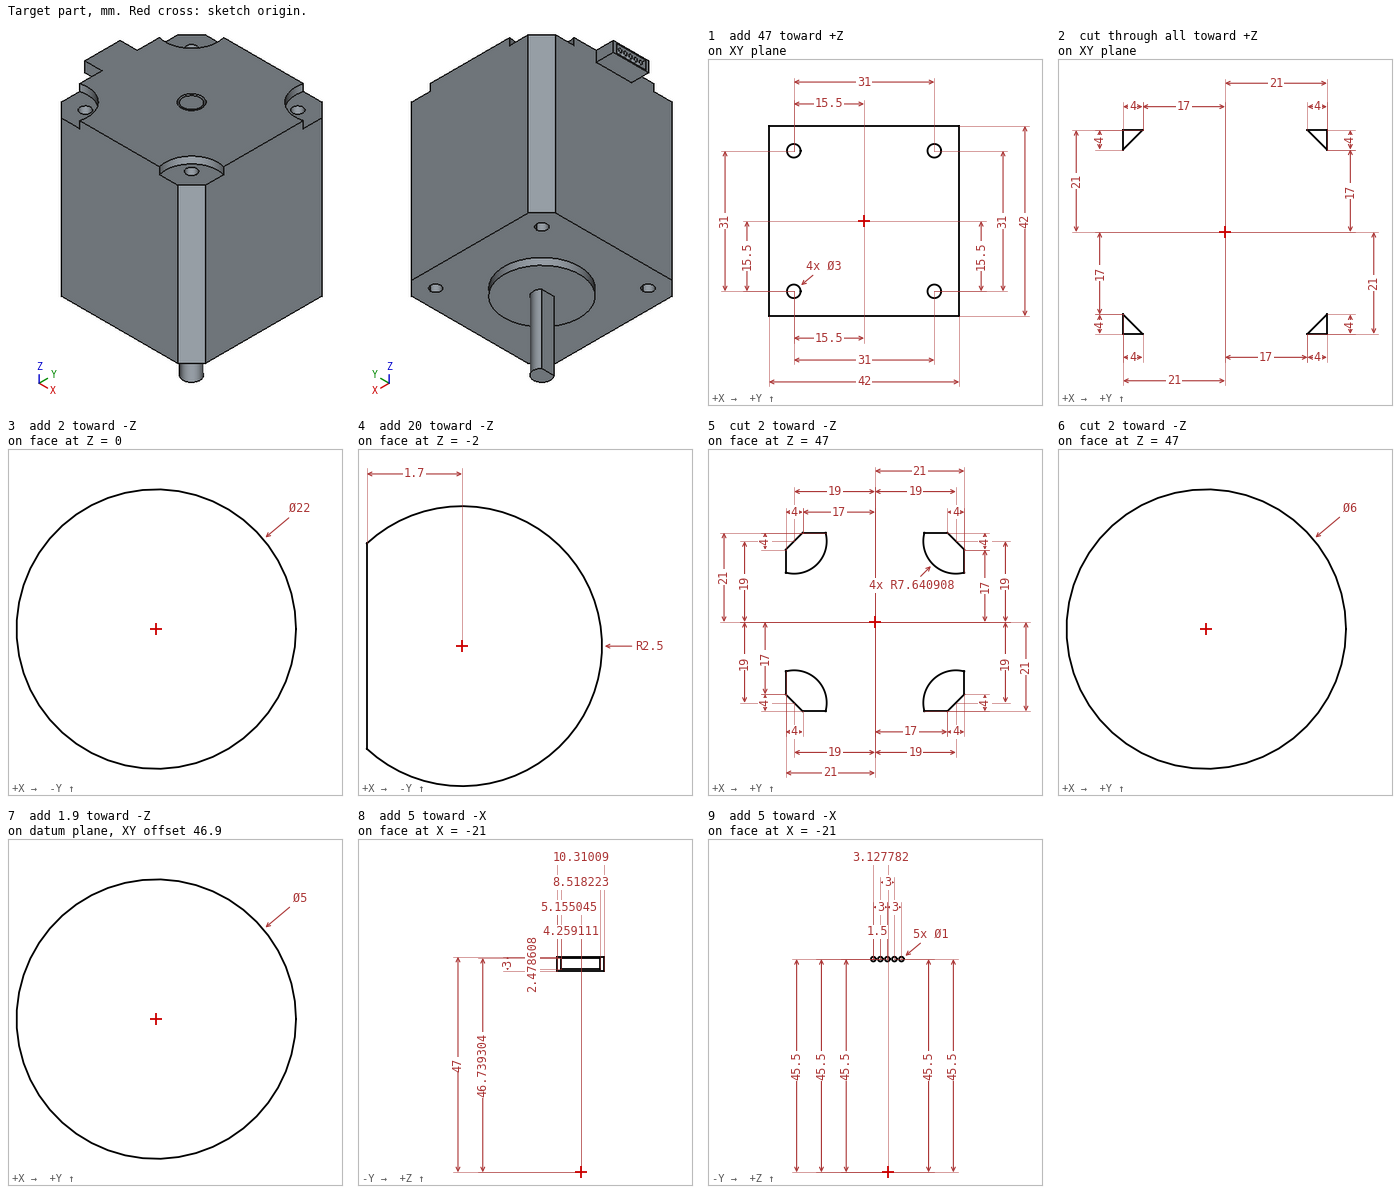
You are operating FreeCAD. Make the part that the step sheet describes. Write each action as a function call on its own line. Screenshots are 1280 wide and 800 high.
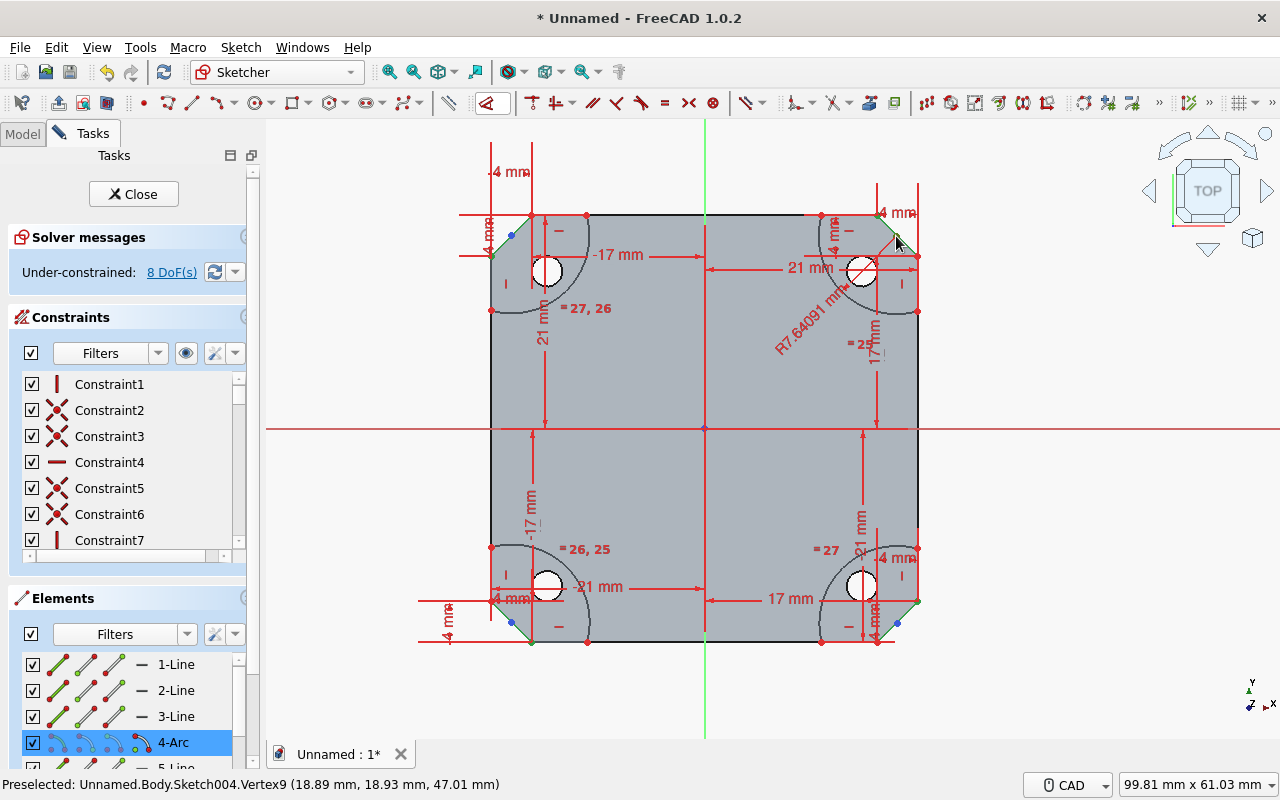
click(504, 104)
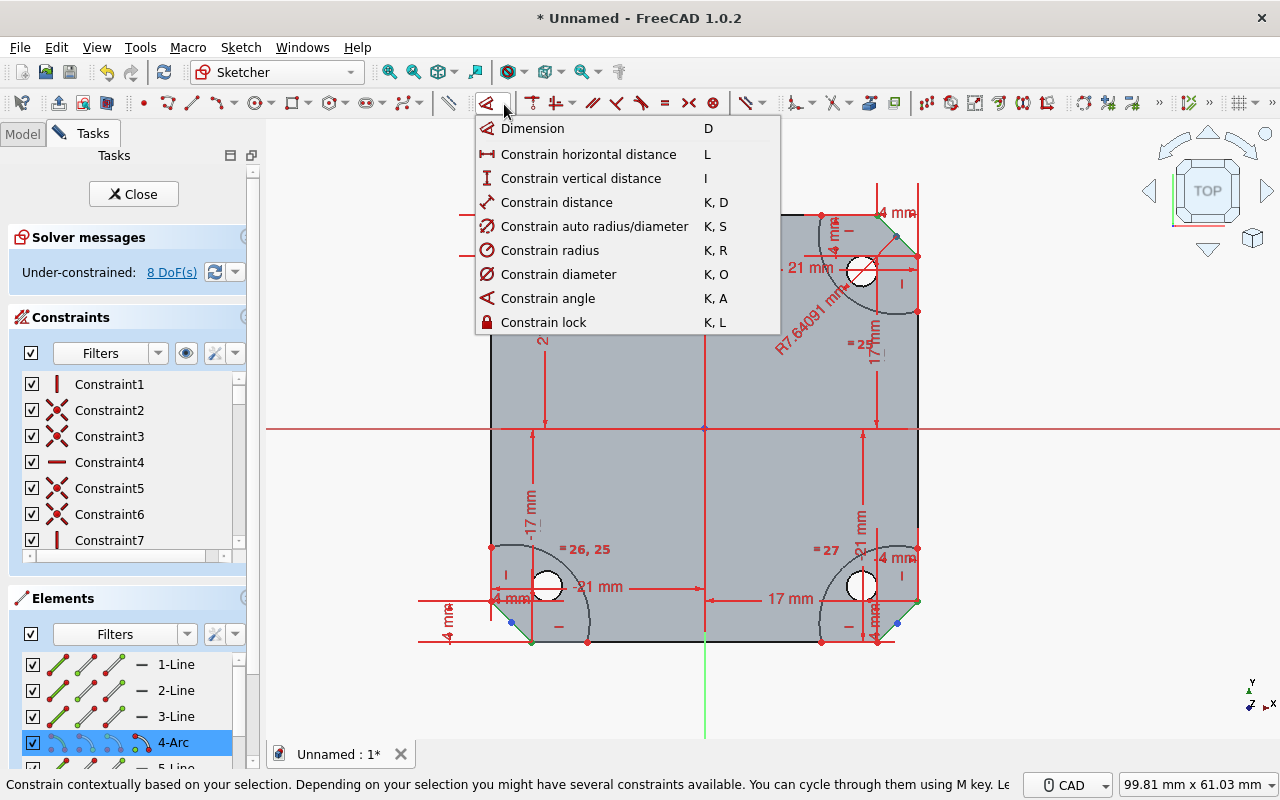
click(628, 154)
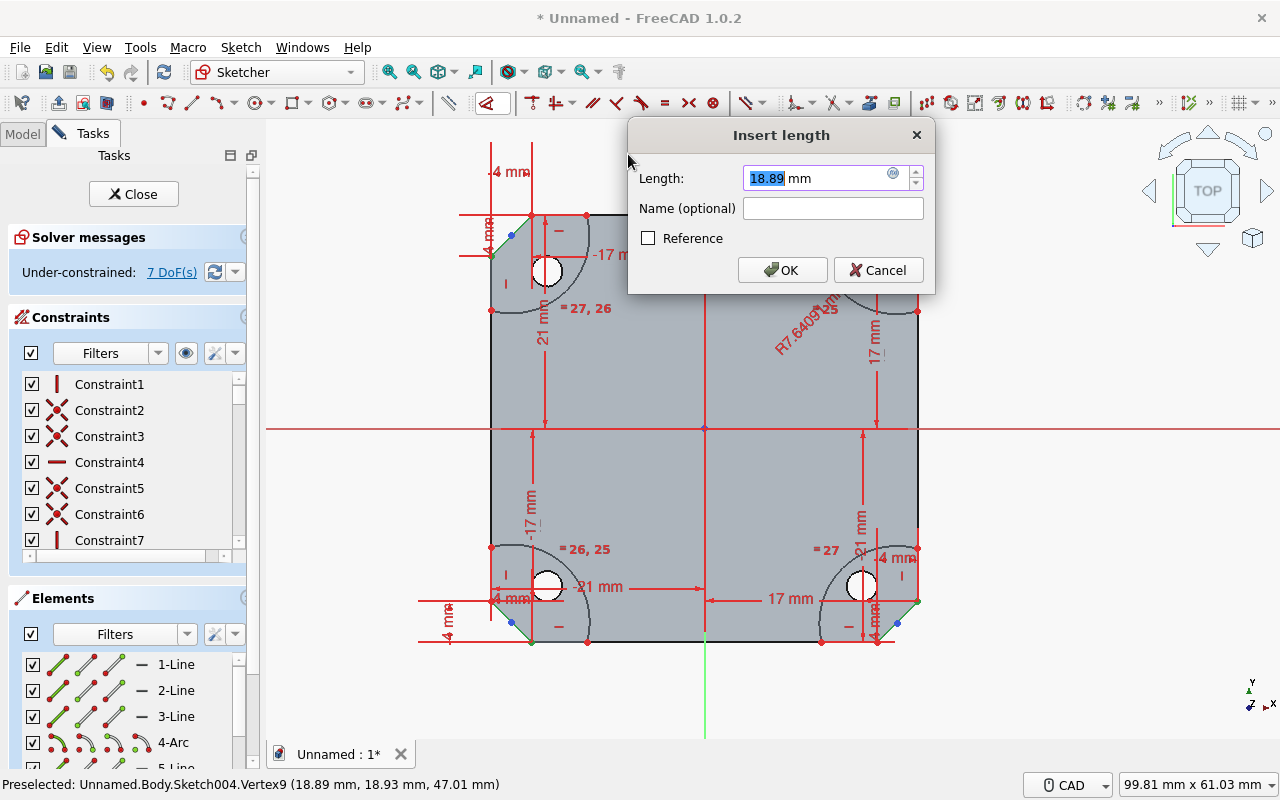
text(19)
key(Return)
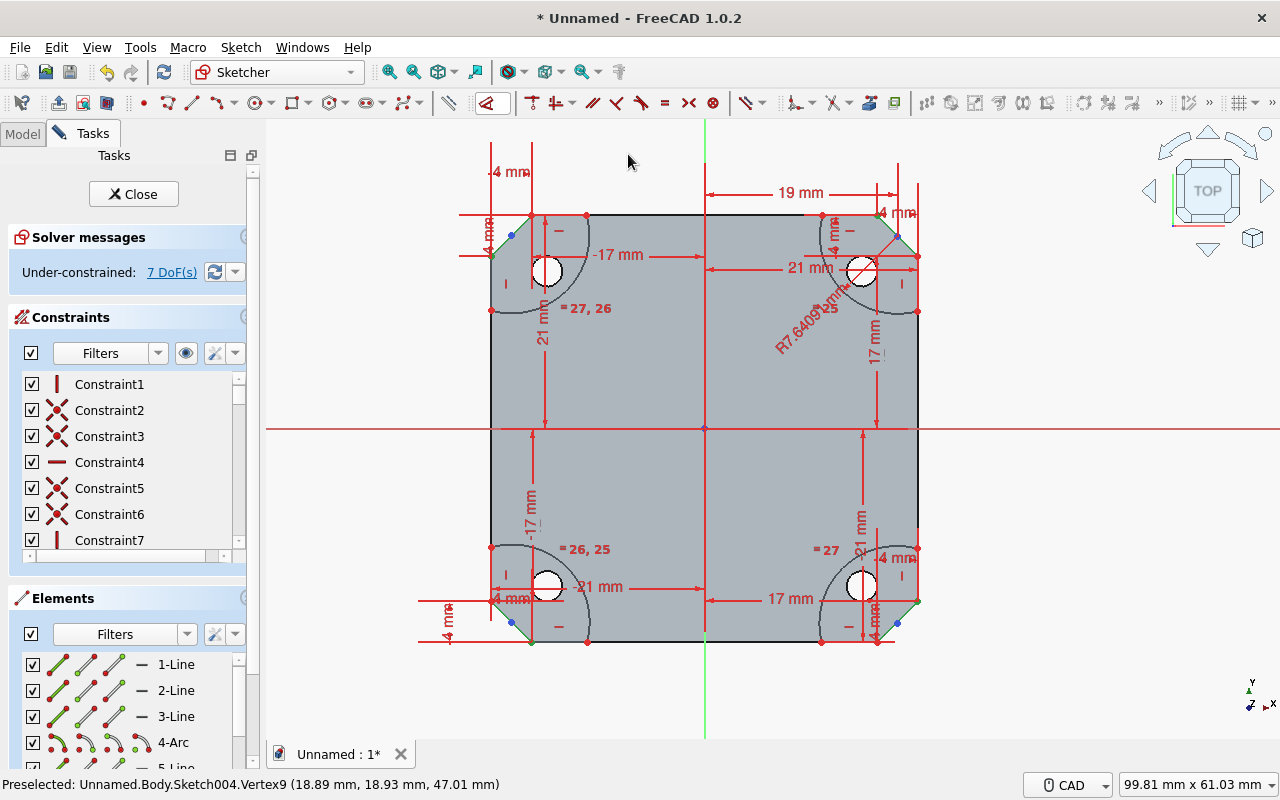
click(898, 236)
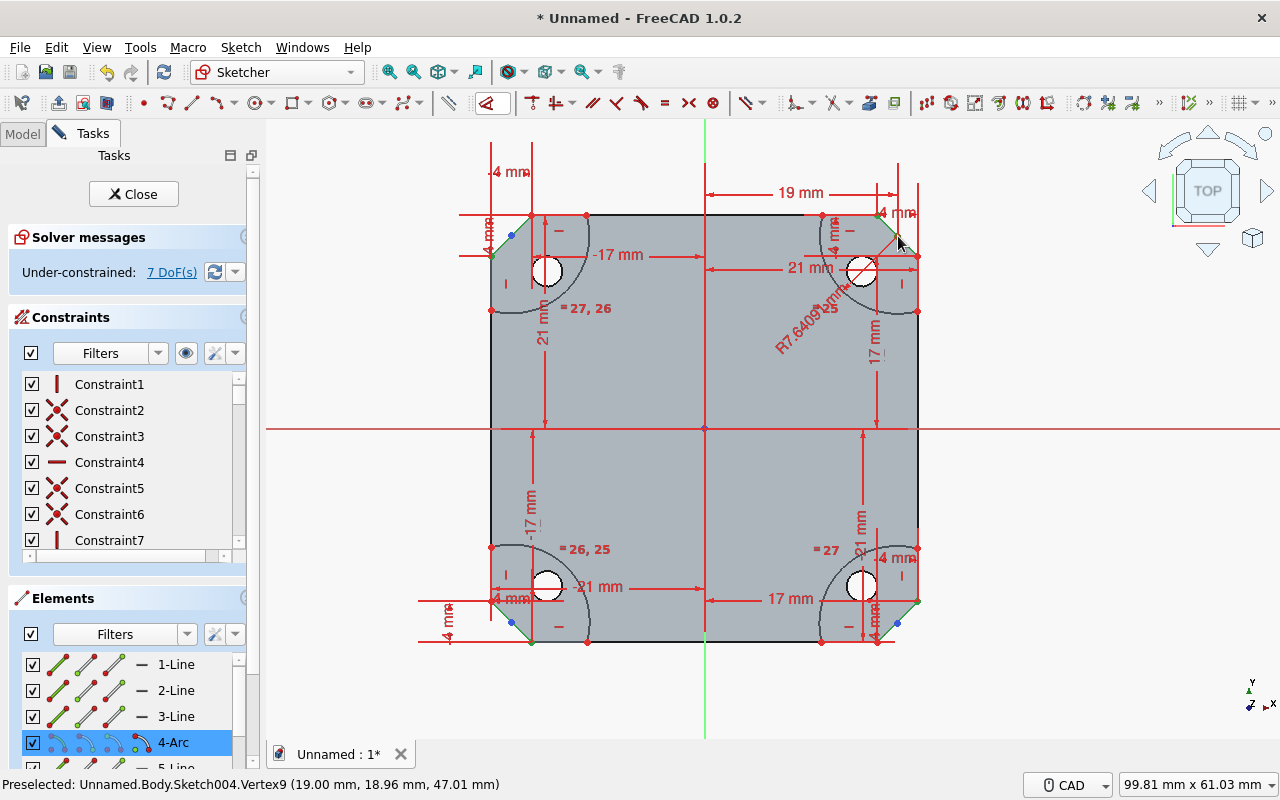
click(504, 104)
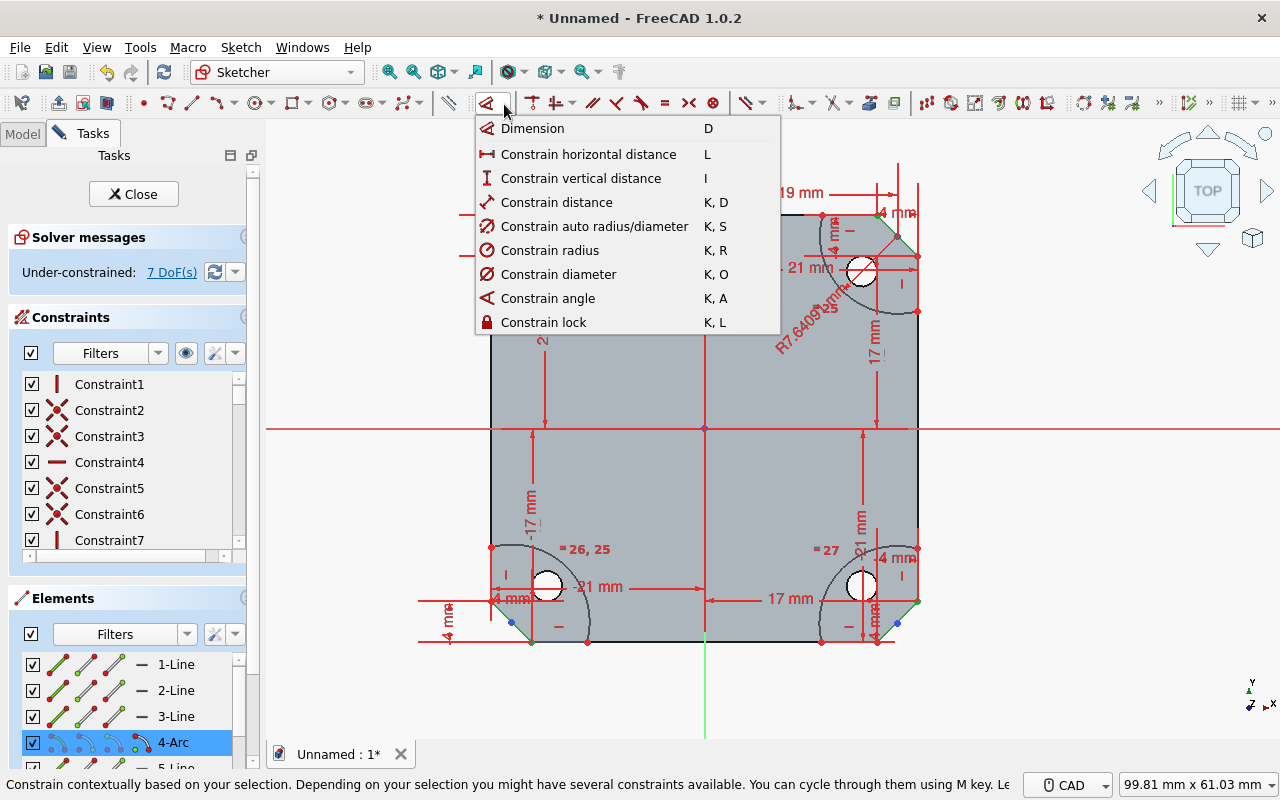
click(628, 178)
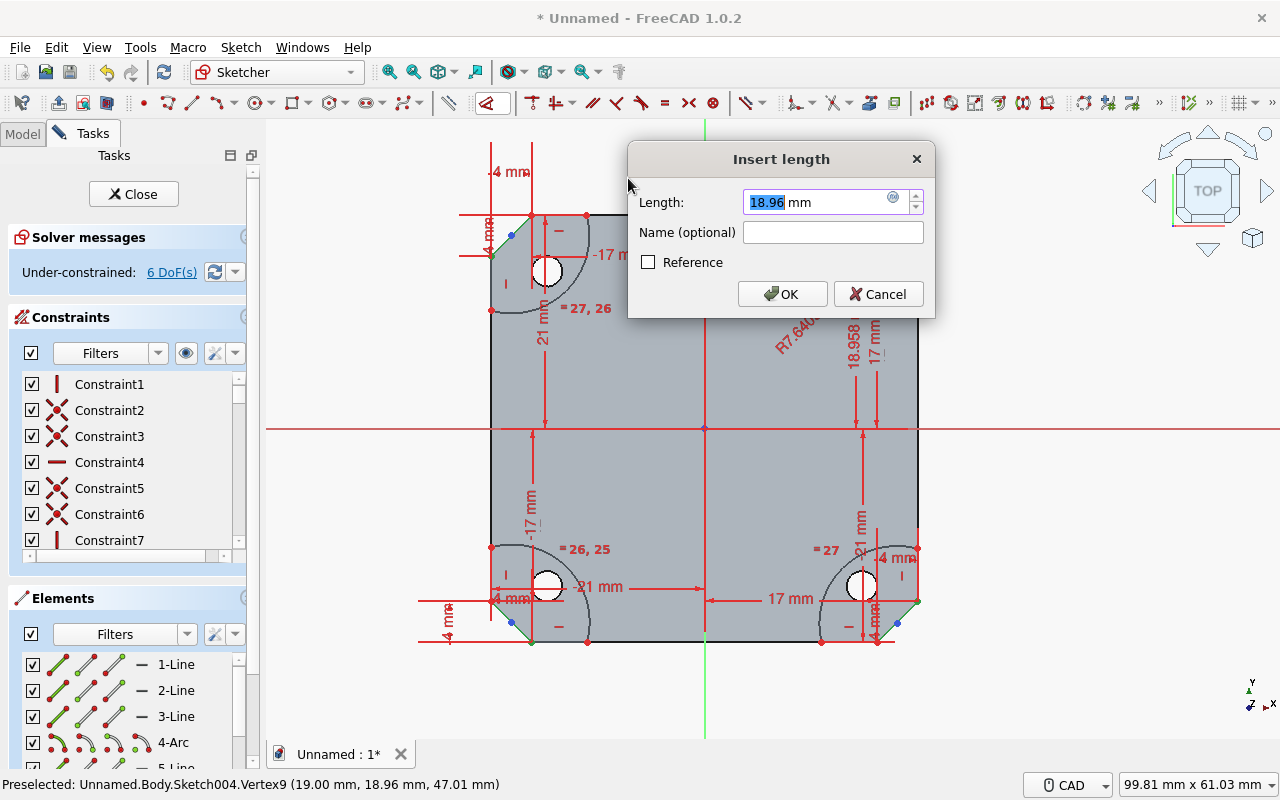
text(19)
key(Return)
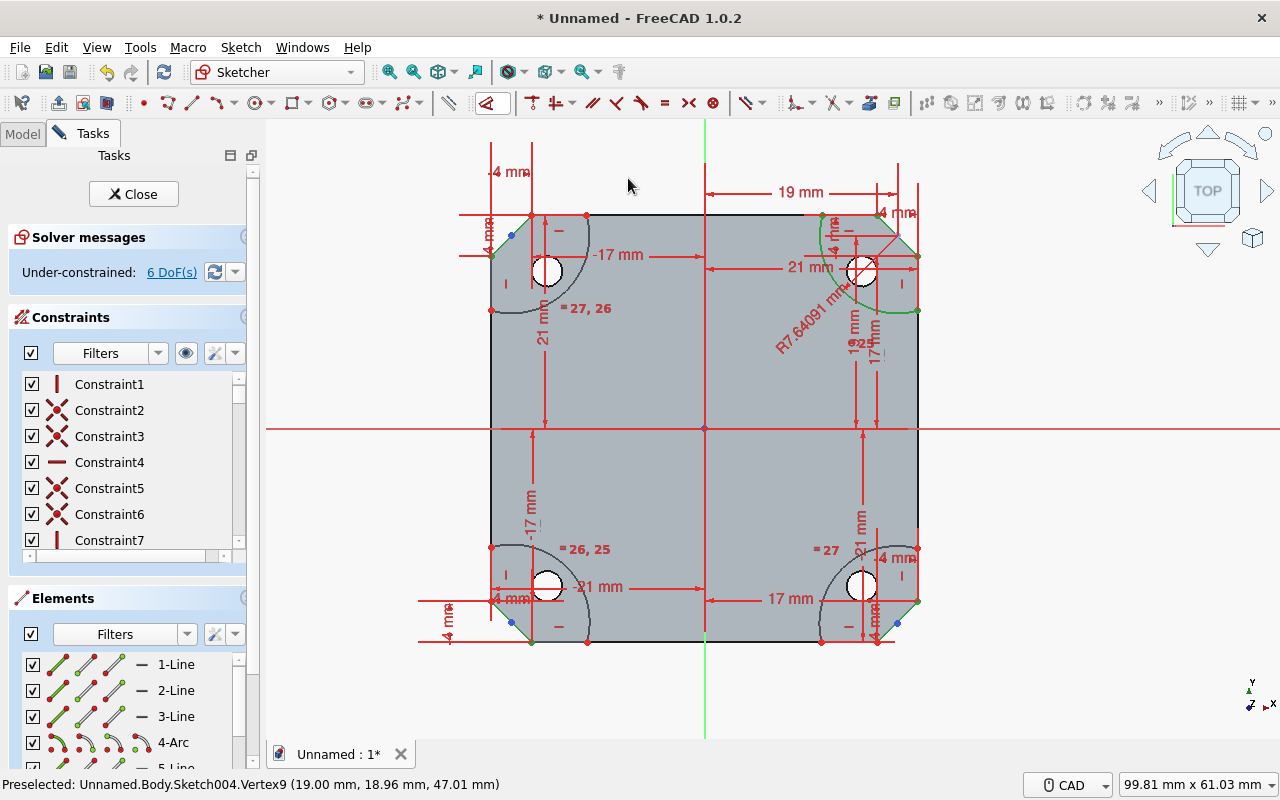
click(512, 622)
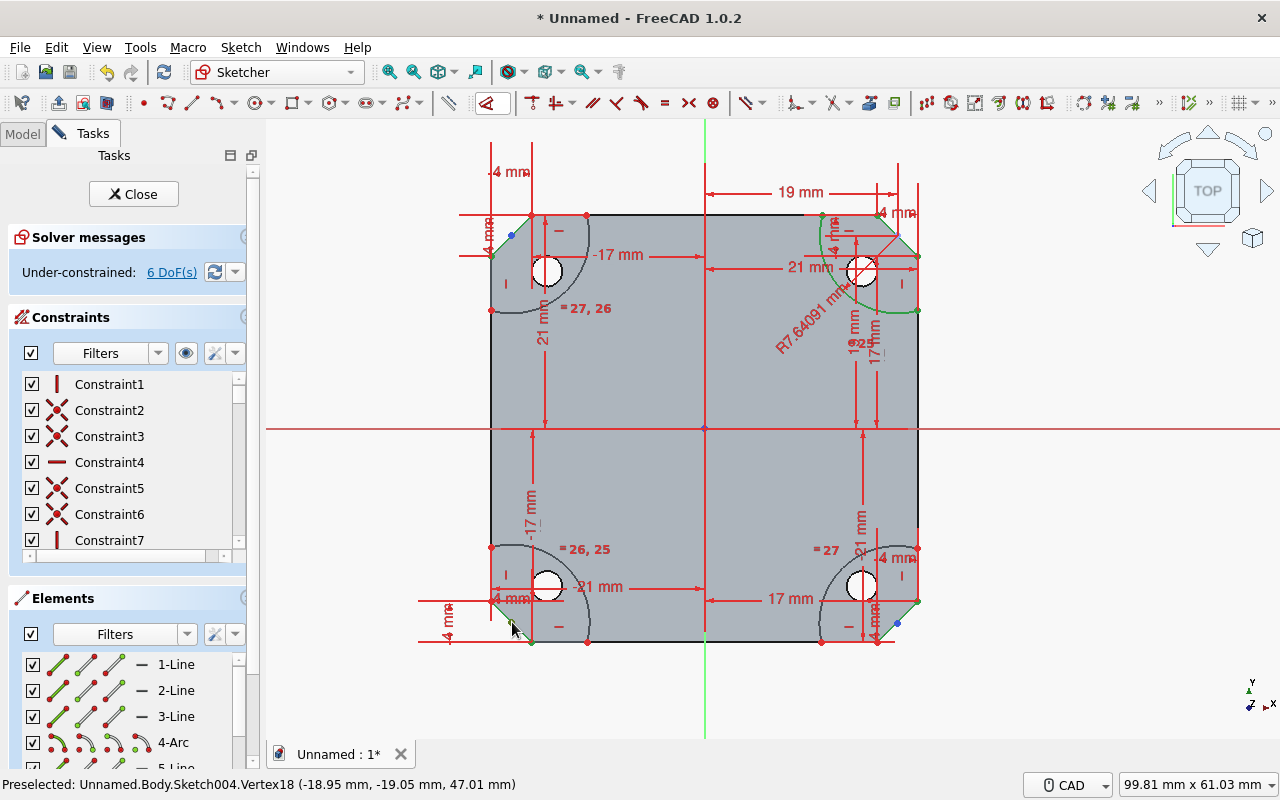
click(504, 104)